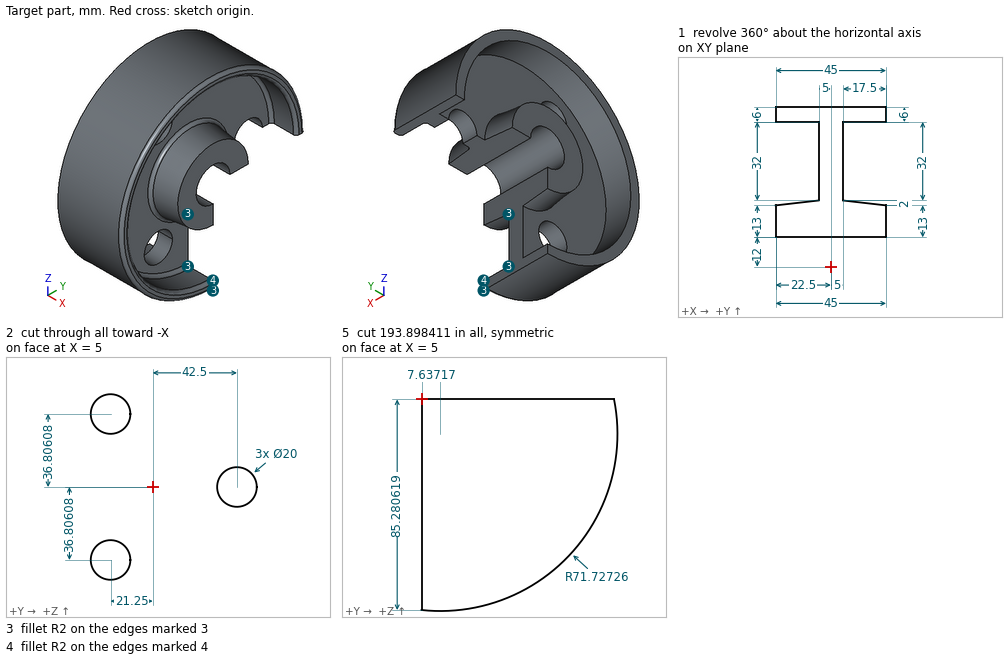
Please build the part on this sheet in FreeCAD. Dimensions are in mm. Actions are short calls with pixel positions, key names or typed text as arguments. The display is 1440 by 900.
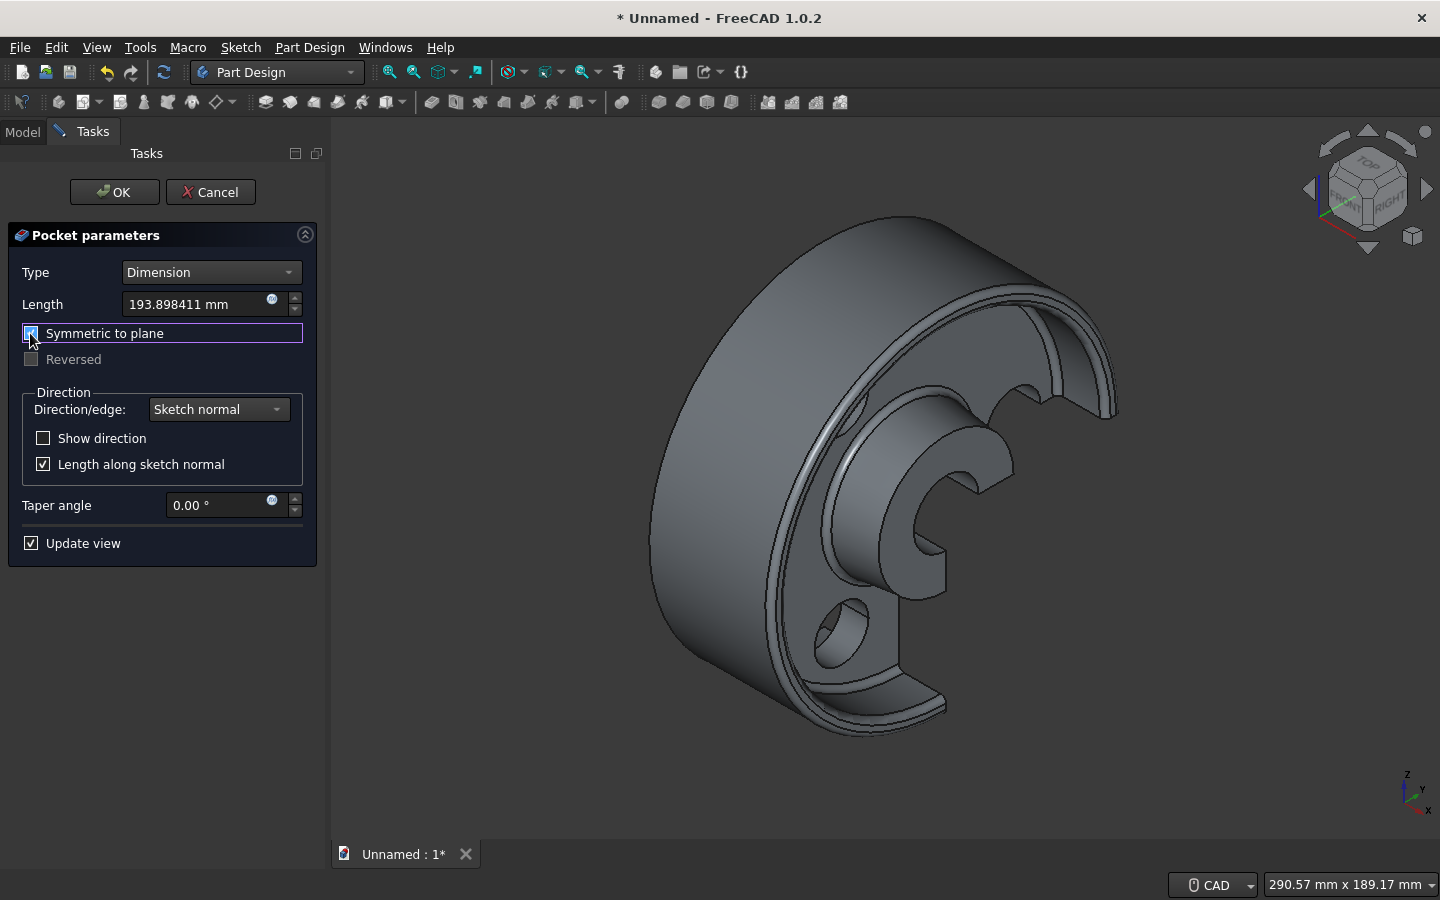
click(115, 192)